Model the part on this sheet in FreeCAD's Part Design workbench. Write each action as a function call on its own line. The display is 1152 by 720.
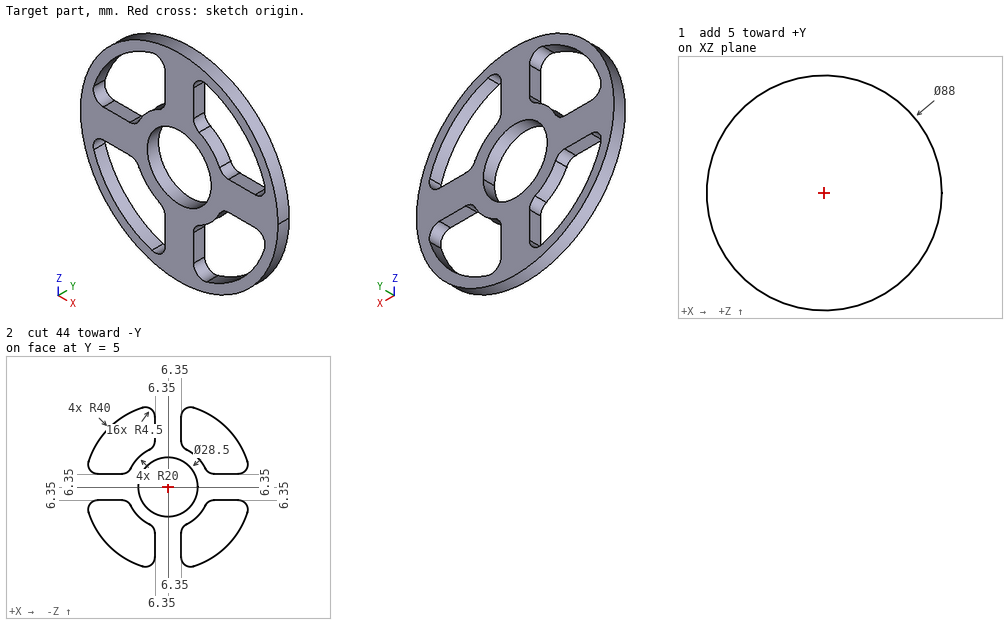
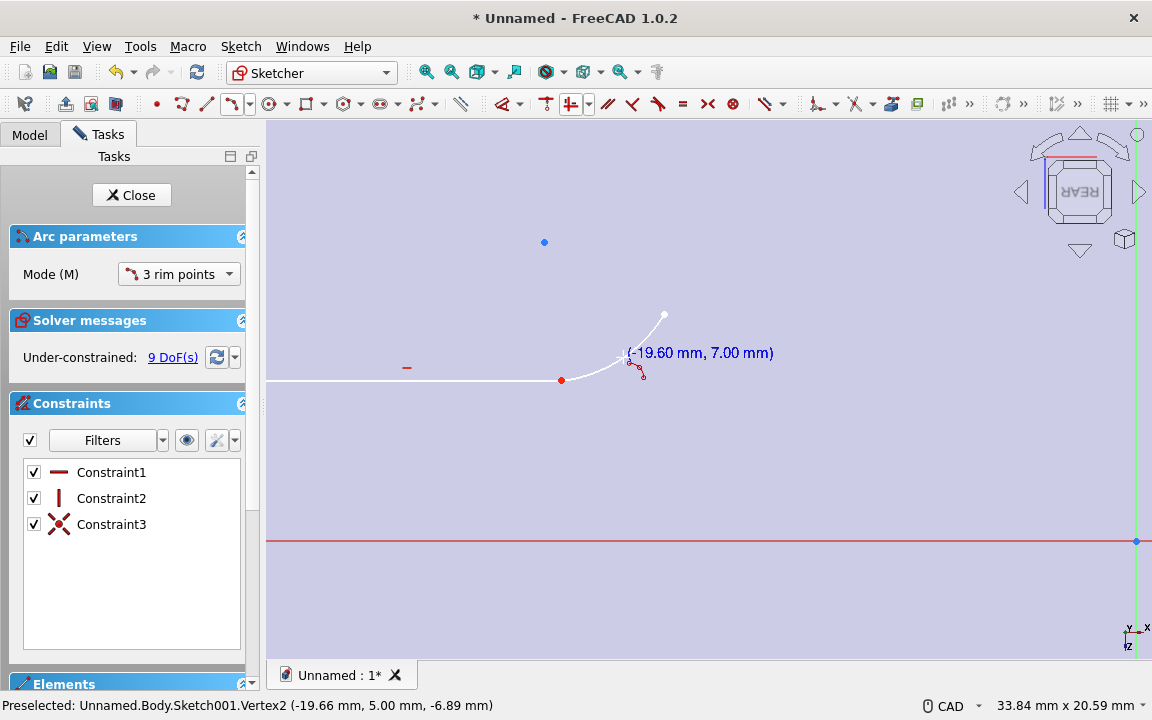
scroll(542, 359, down, 9)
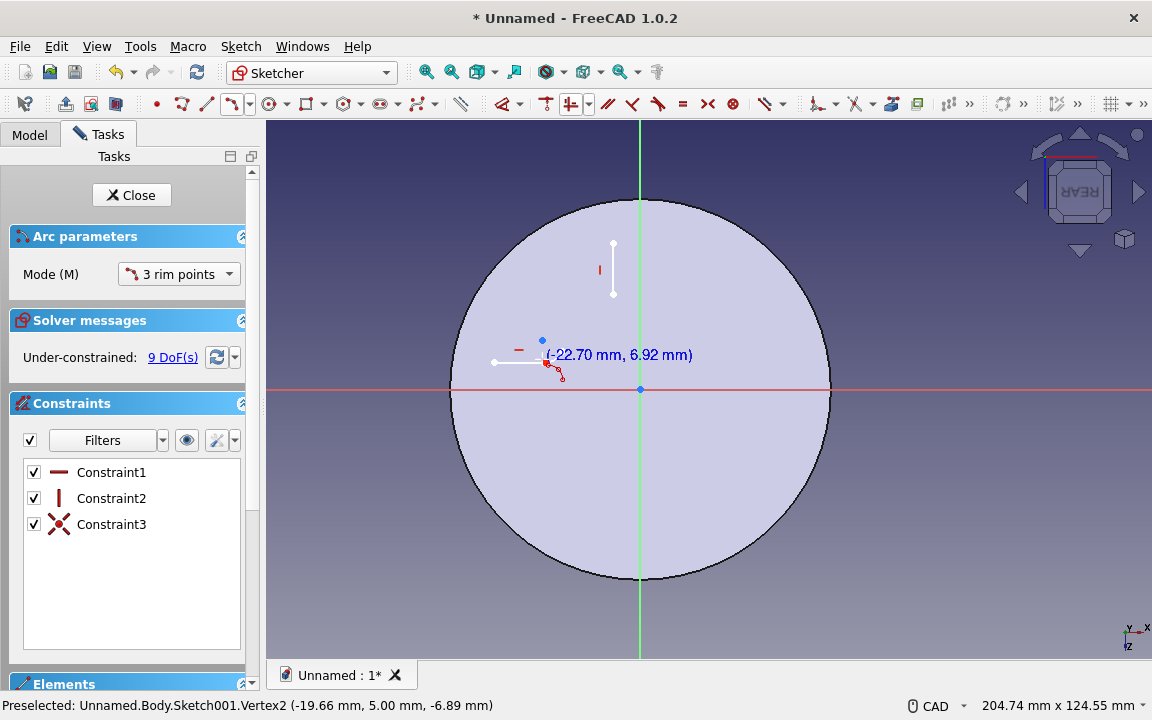
click(562, 352)
click(602, 312)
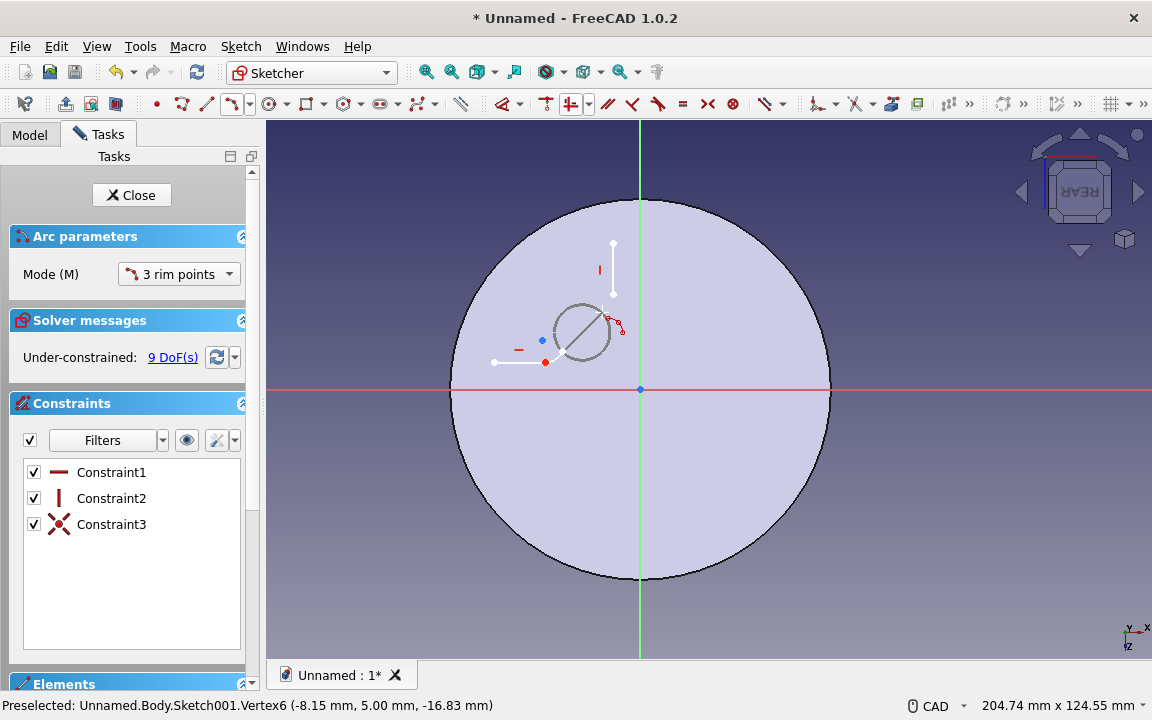
scroll(579, 328, up, 7)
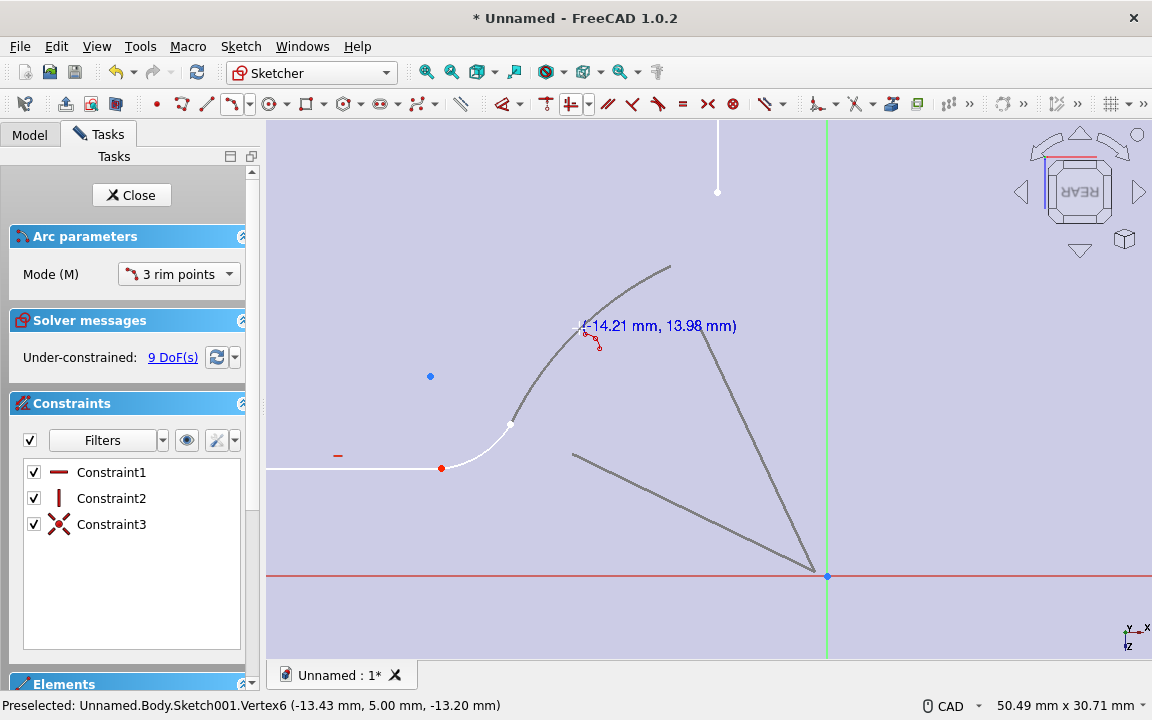
click(579, 328)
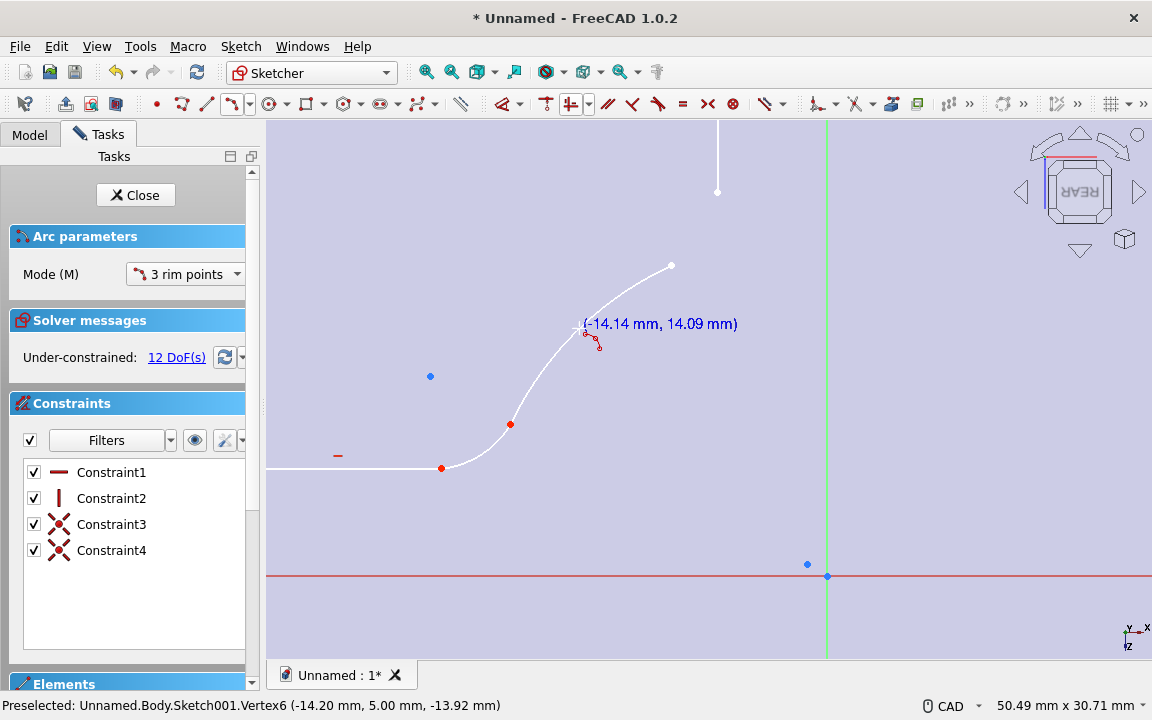
scroll(579, 328, down, 7)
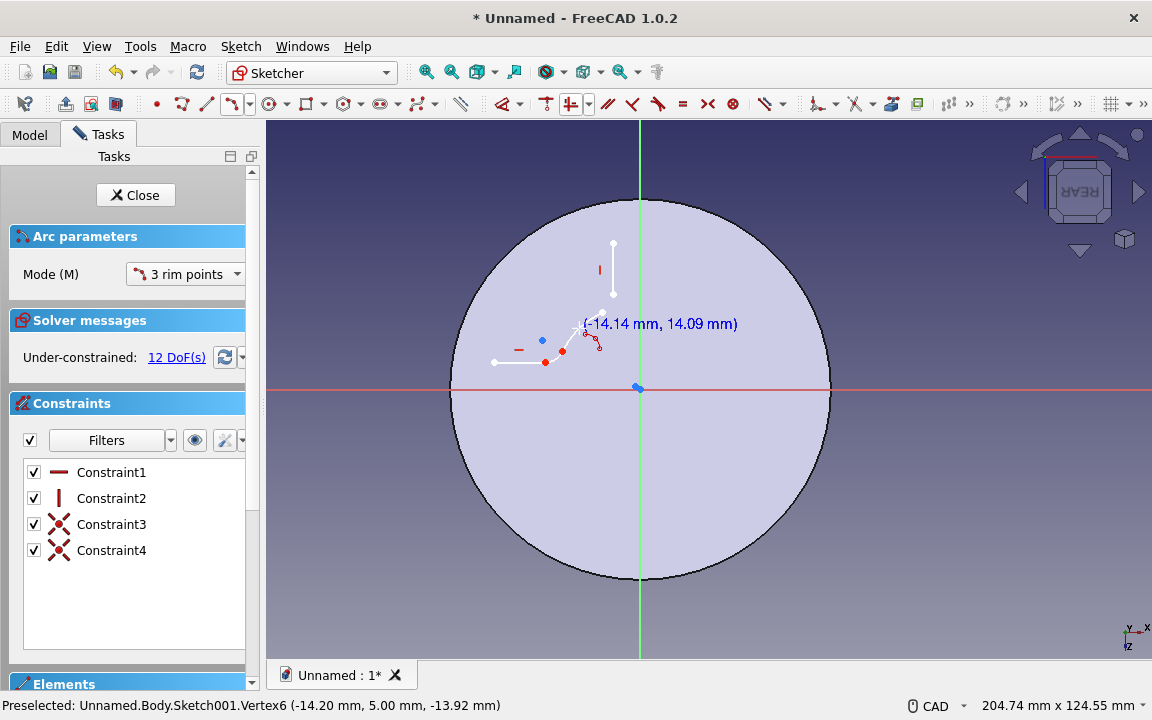
click(602, 313)
click(613, 295)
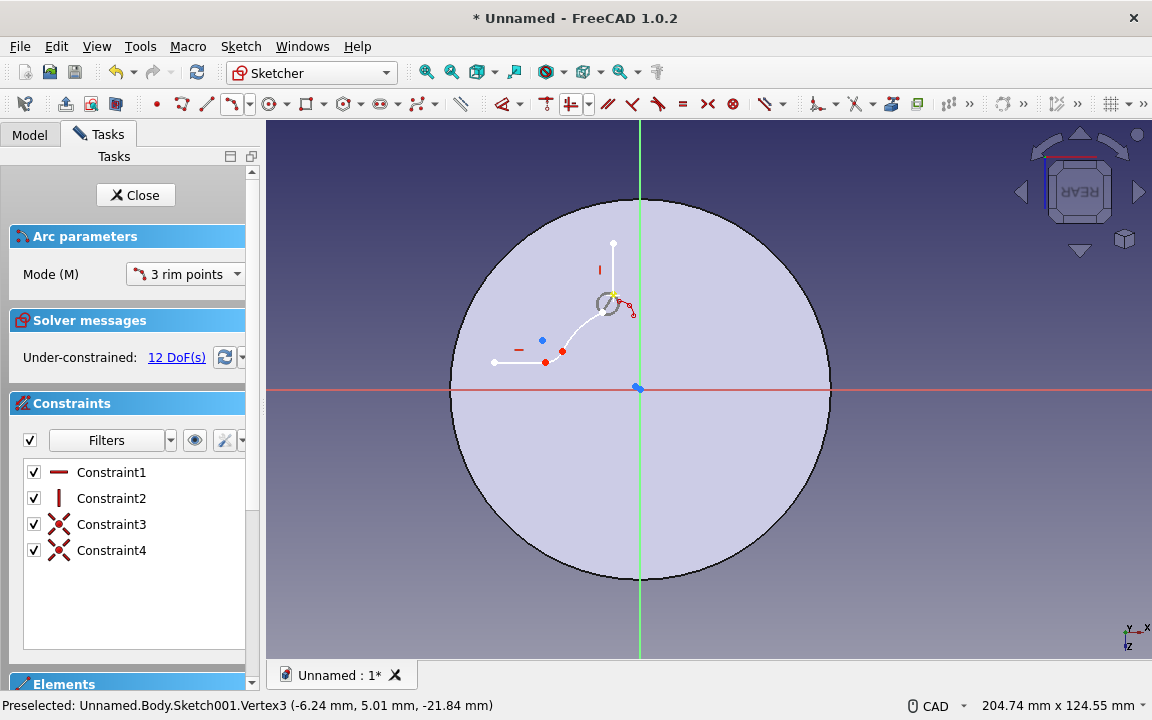
scroll(610, 305, up, 9)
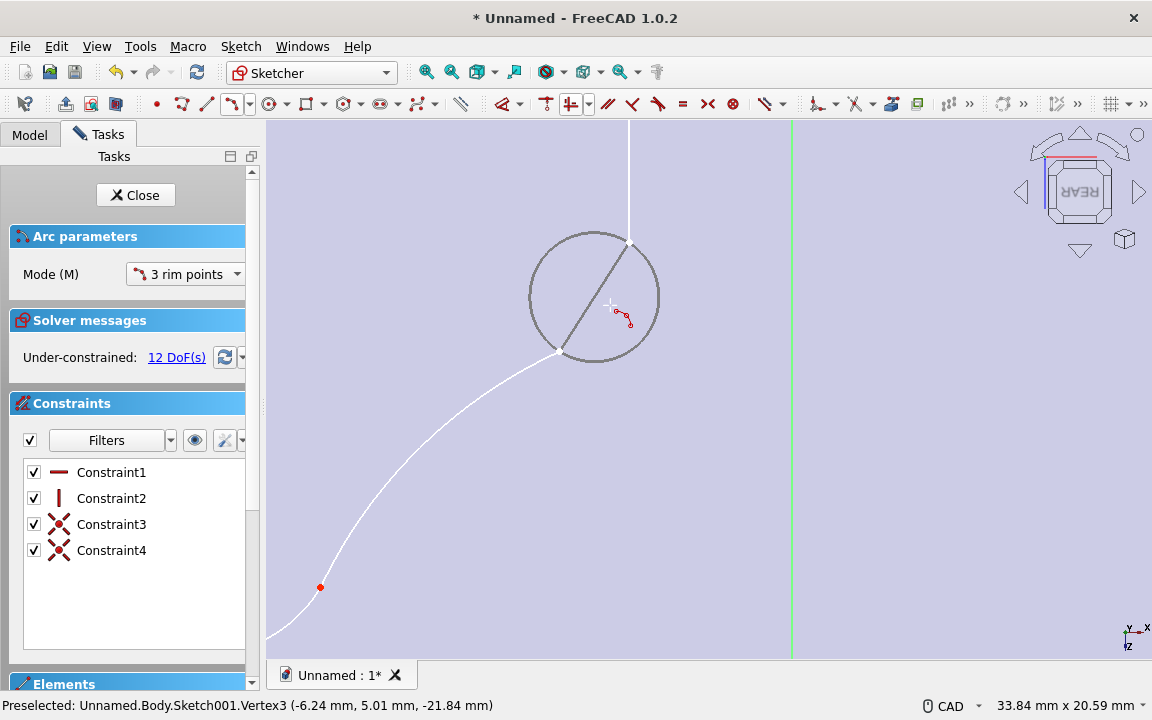
click(608, 302)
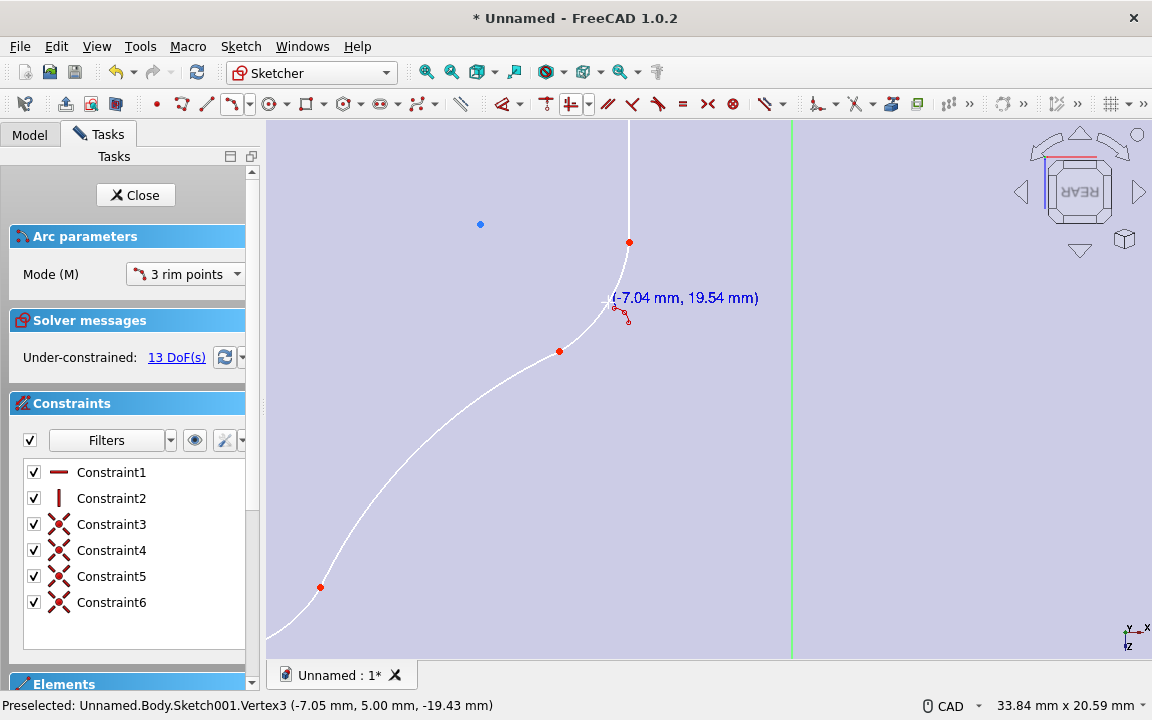
scroll(610, 305, down, 9)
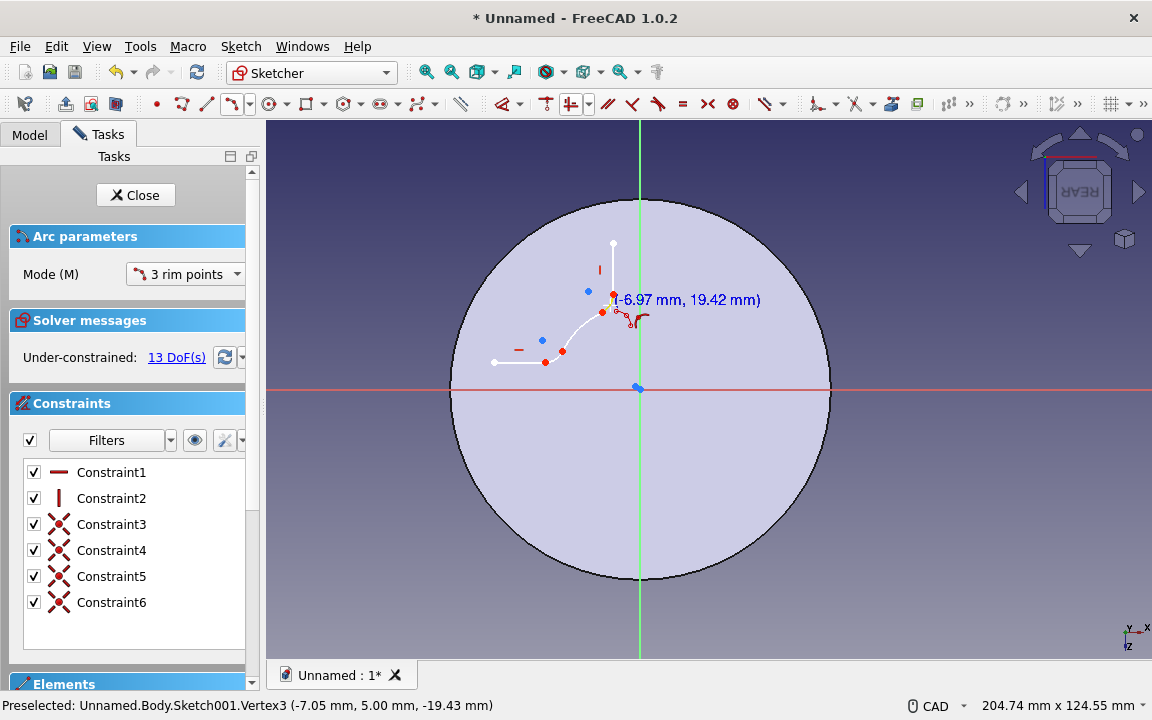
click(613, 244)
click(588, 225)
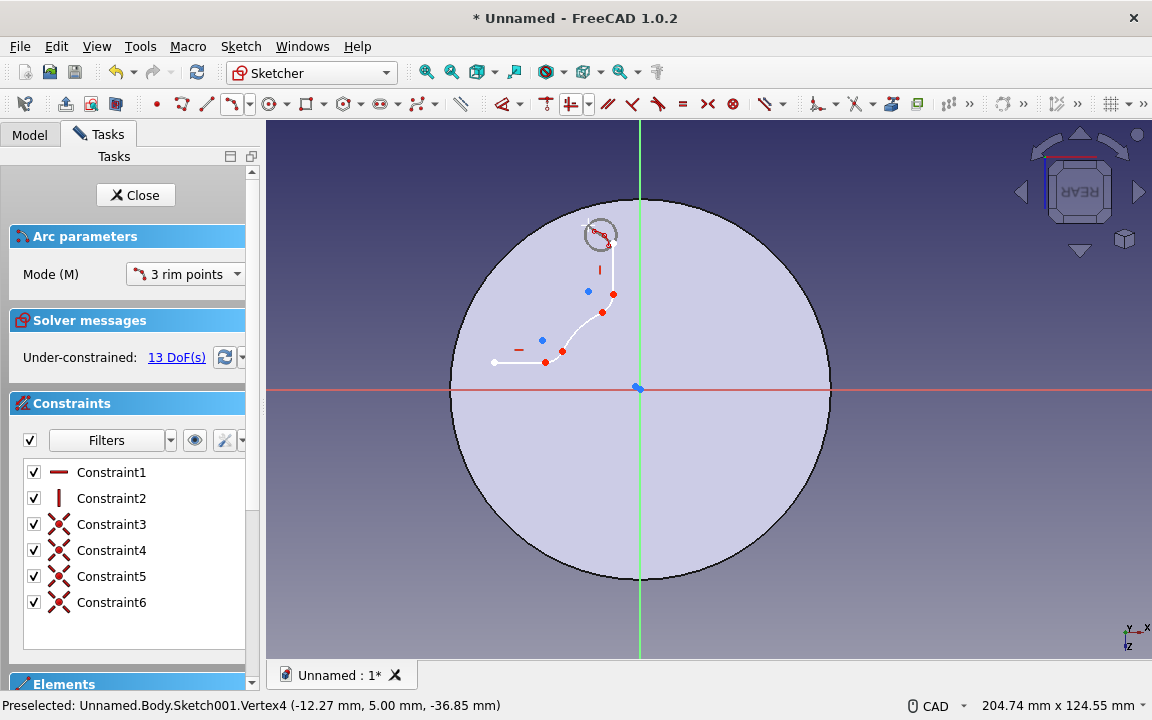
scroll(605, 227, up, 4)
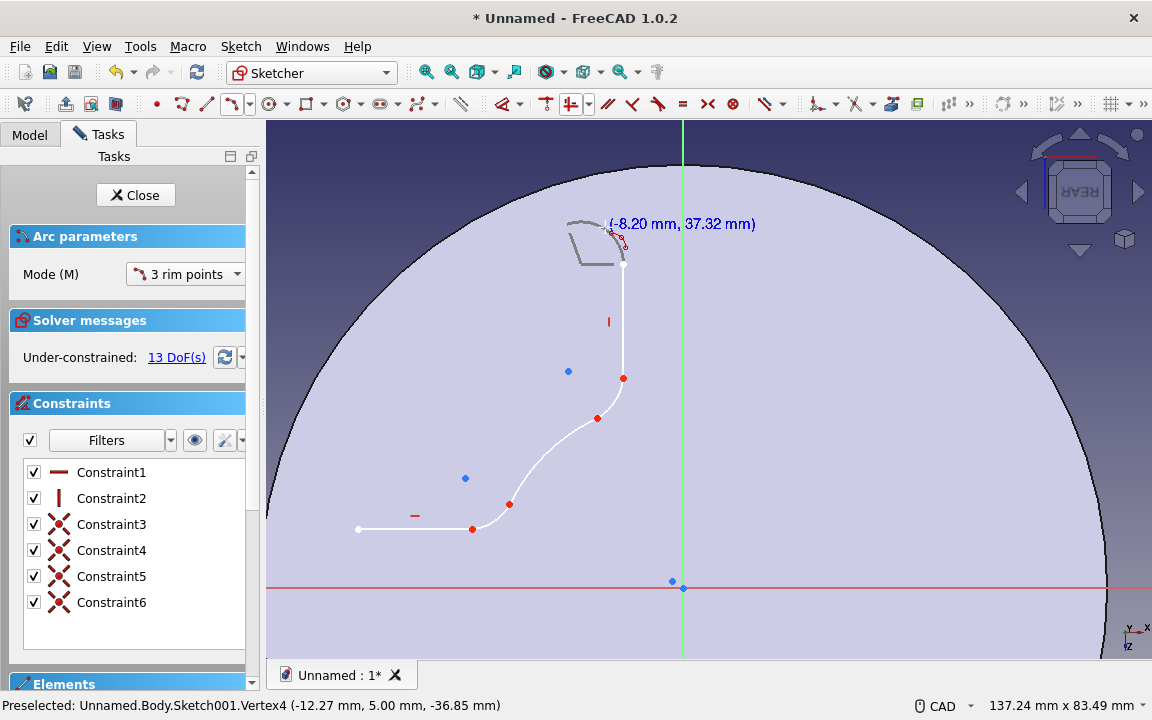
click(605, 228)